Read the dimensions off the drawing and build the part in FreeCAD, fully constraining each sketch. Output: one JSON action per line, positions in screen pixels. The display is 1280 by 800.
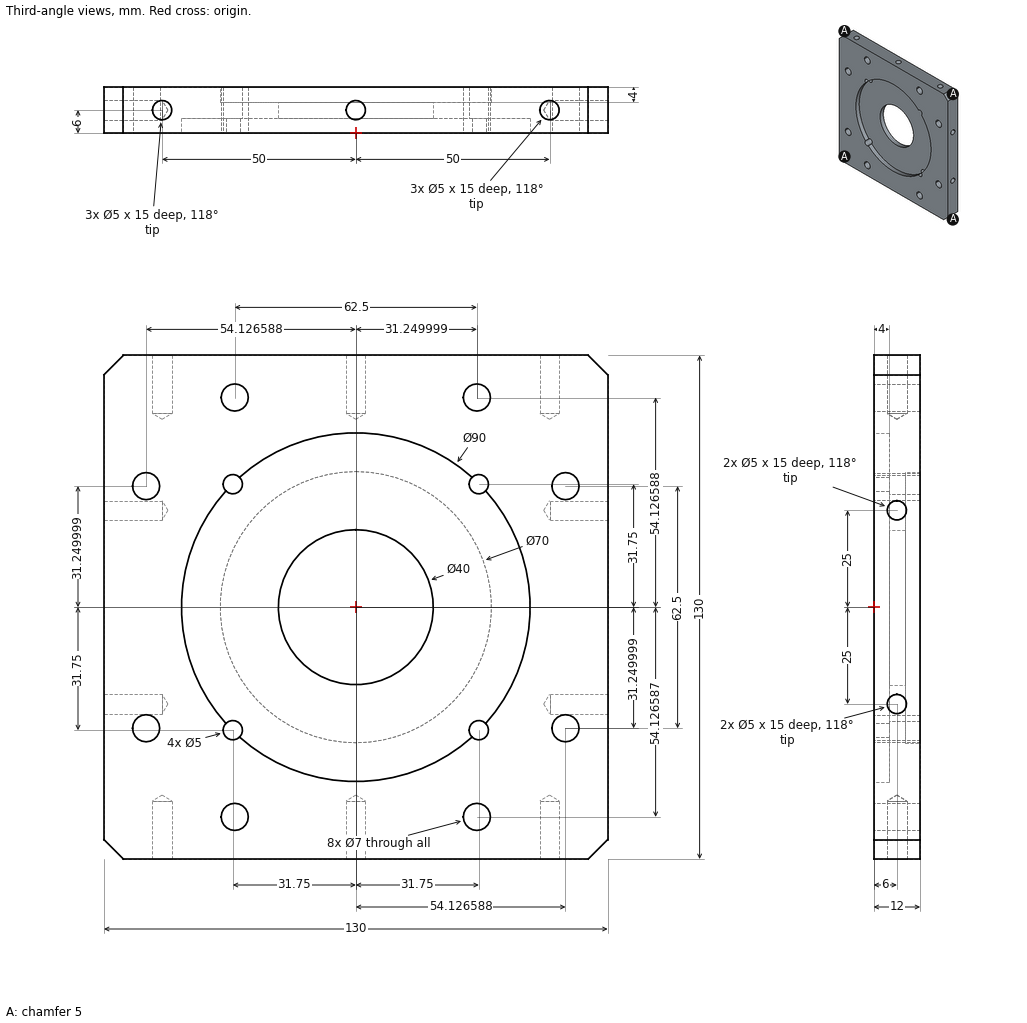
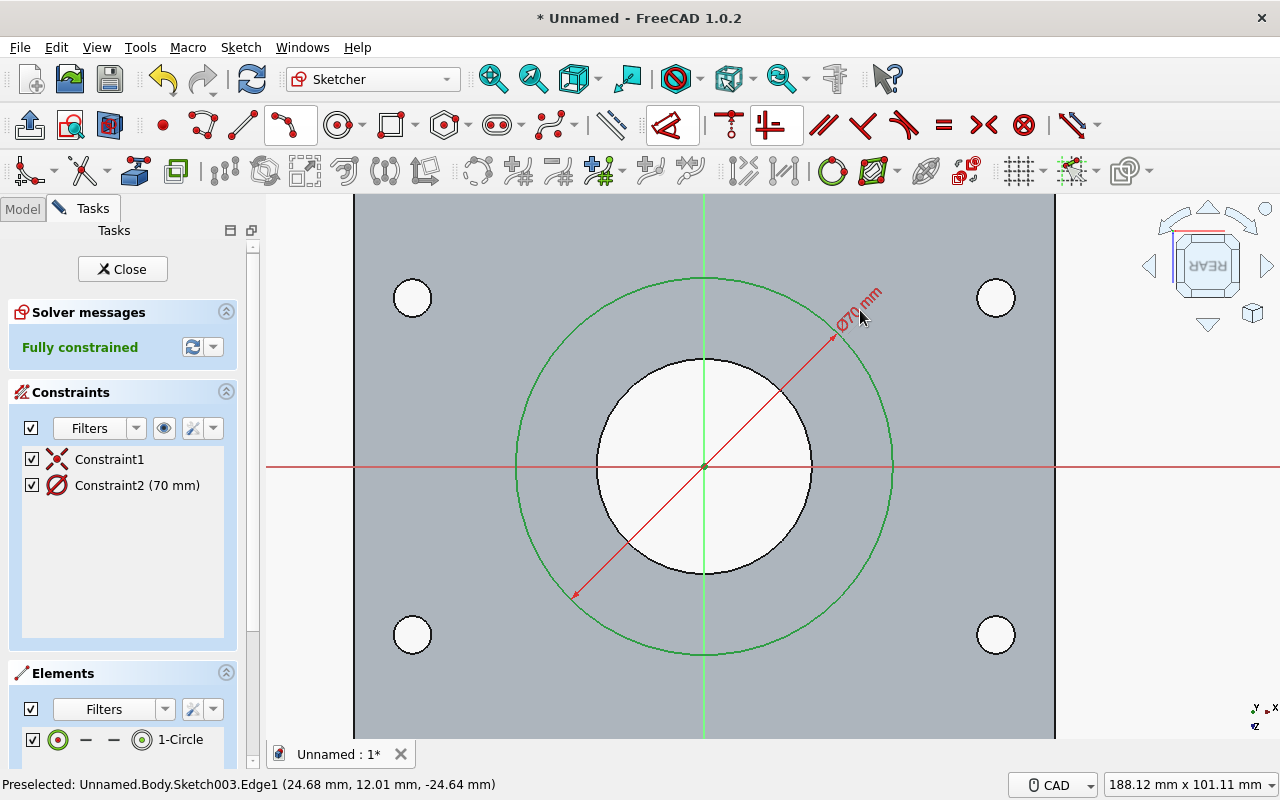
{"action": "left_click", "coordinate": [123, 269]}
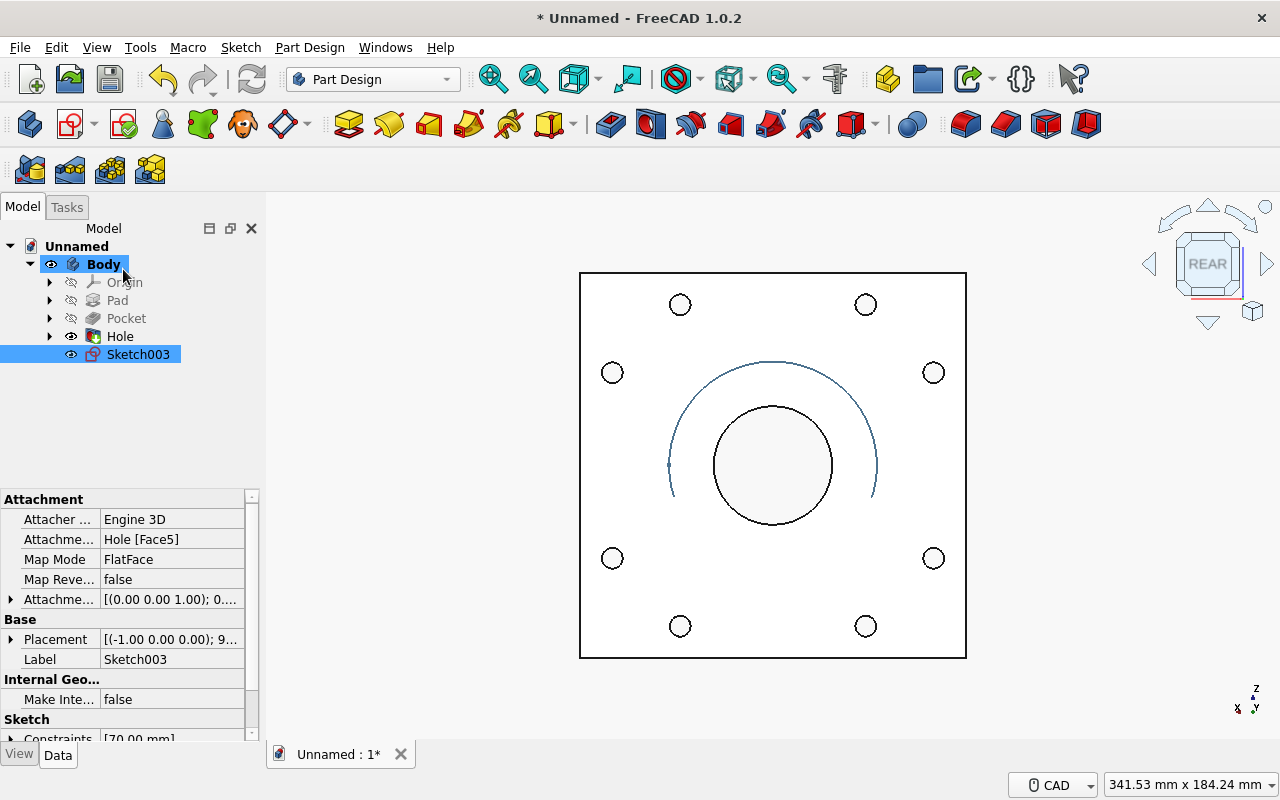
{"action": "left_click", "coordinate": [612, 124]}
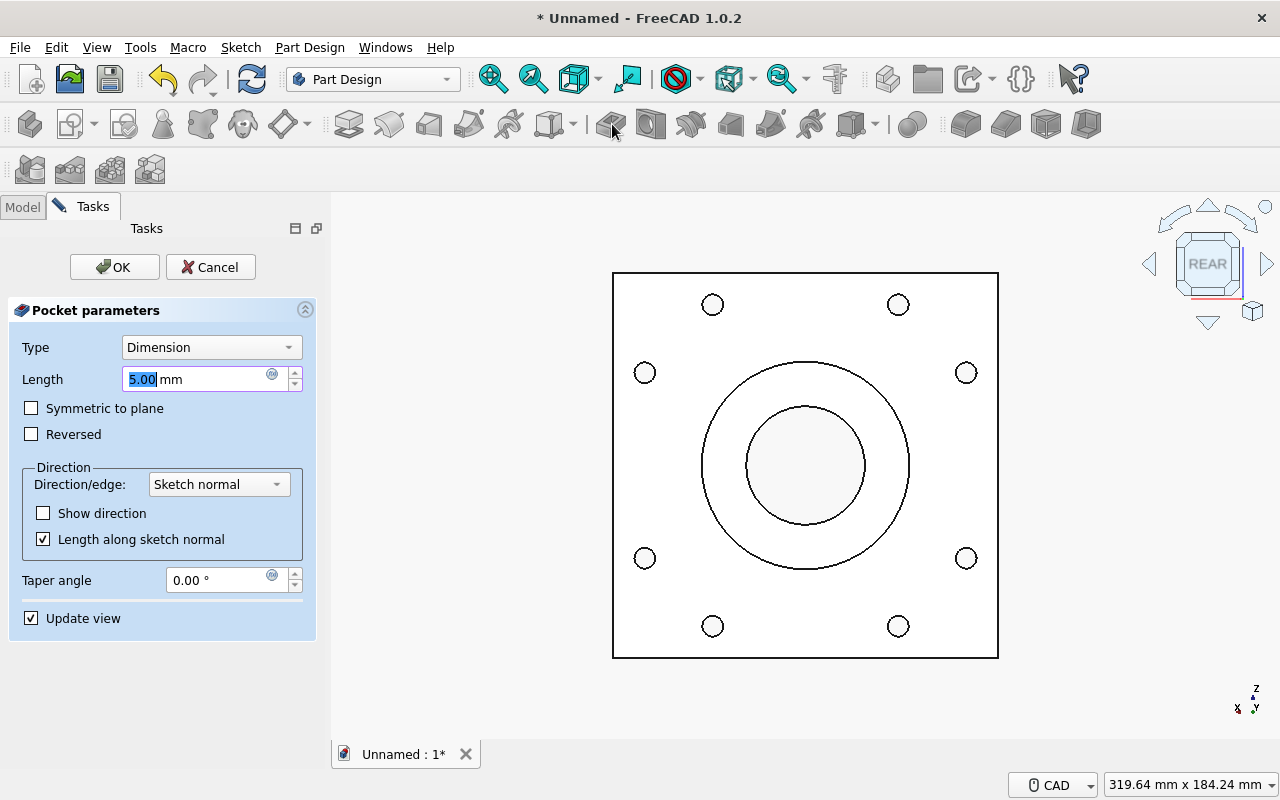
{"action": "type", "text": "4"}
{"action": "key", "text": "Tab"}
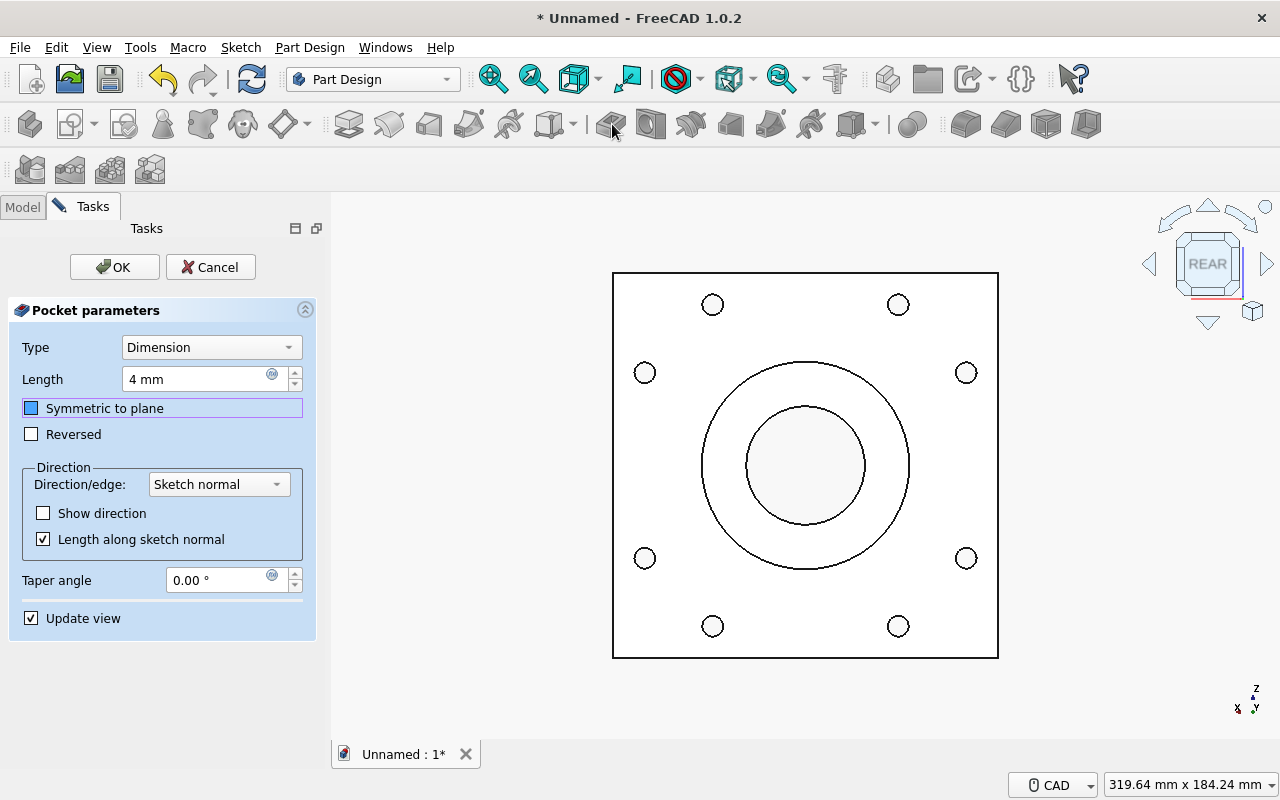
{"action": "left_click", "coordinate": [115, 267]}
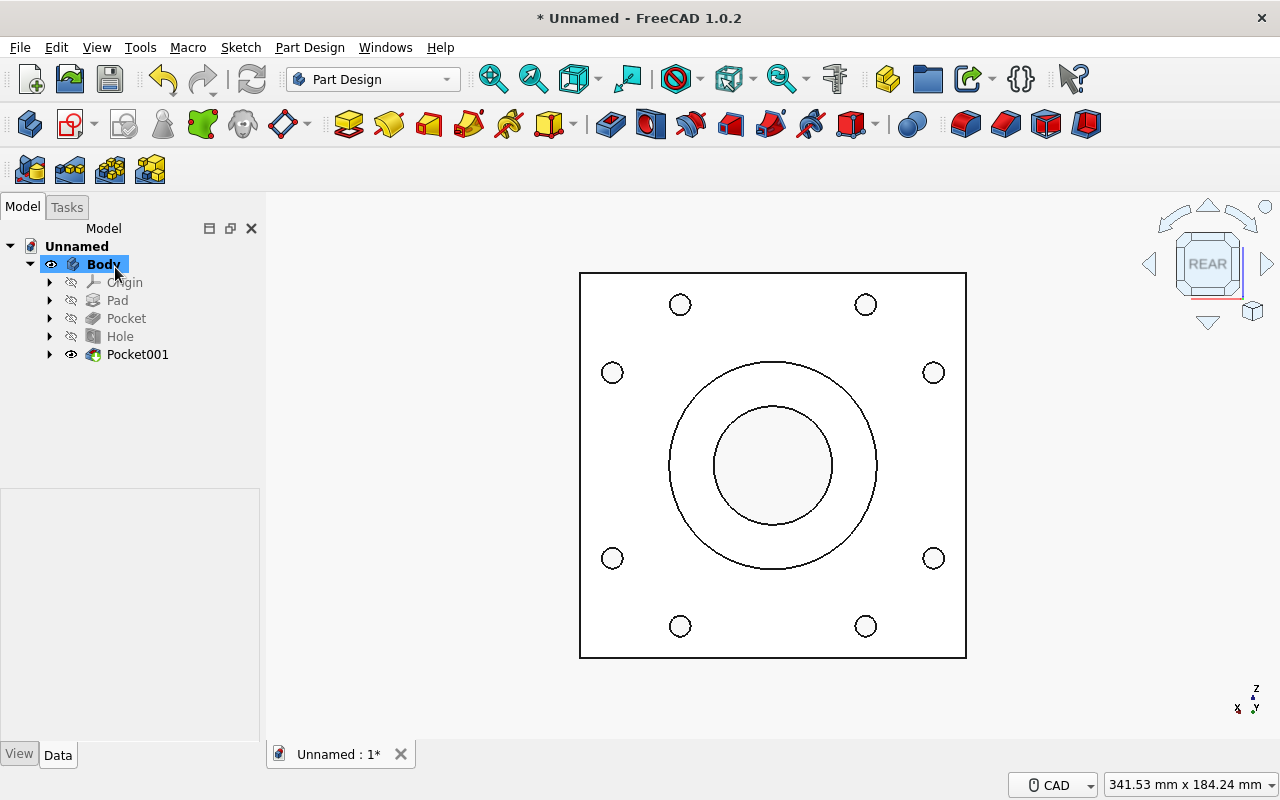
{"action": "key", "text": "0"}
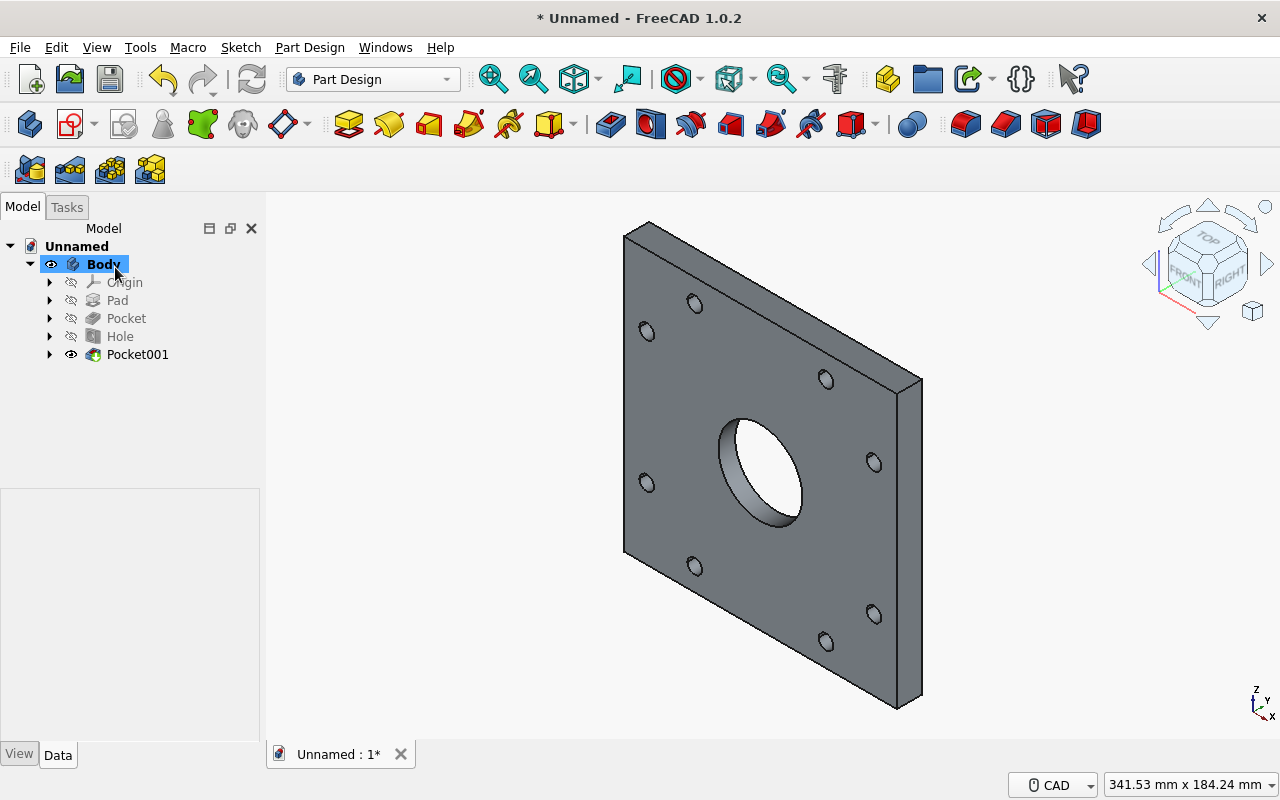
{"action": "left_click", "coordinate": [721, 359]}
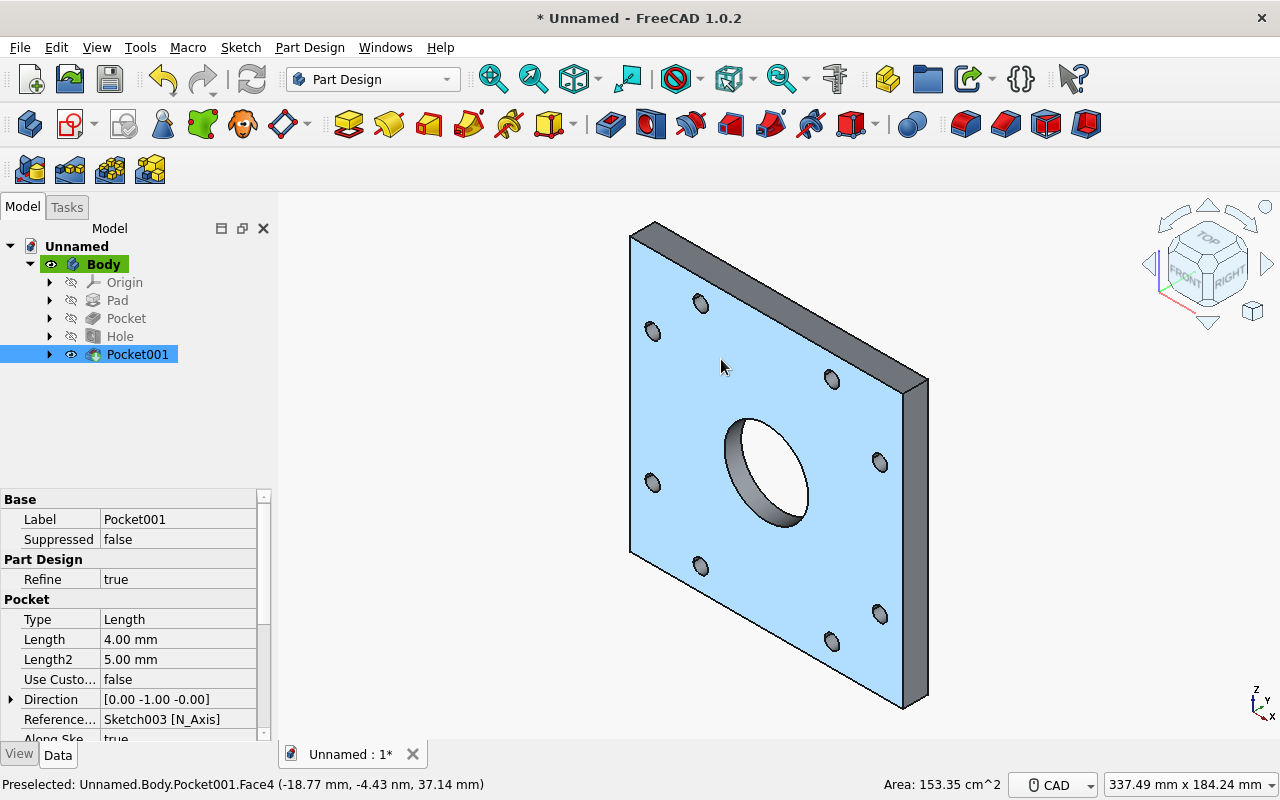
{"action": "left_click", "coordinate": [70, 124]}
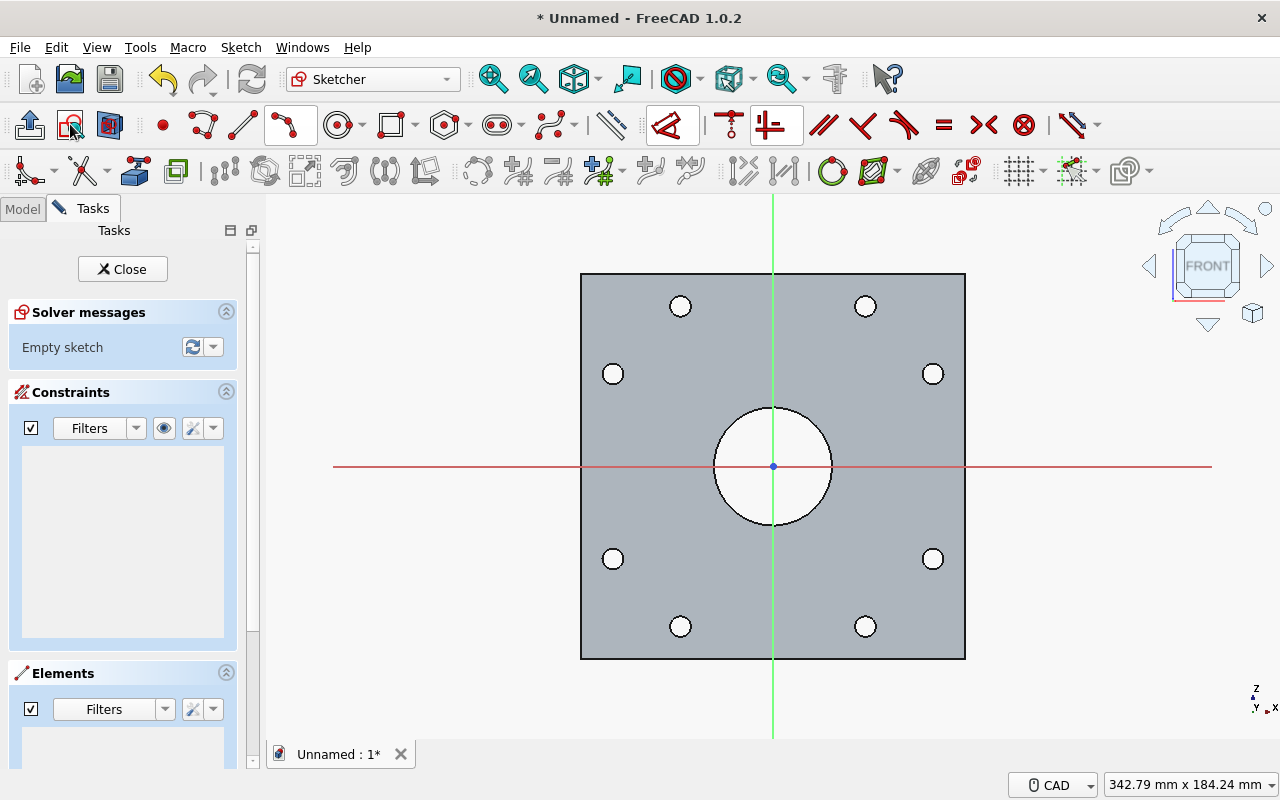
{"action": "key", "text": "g c"}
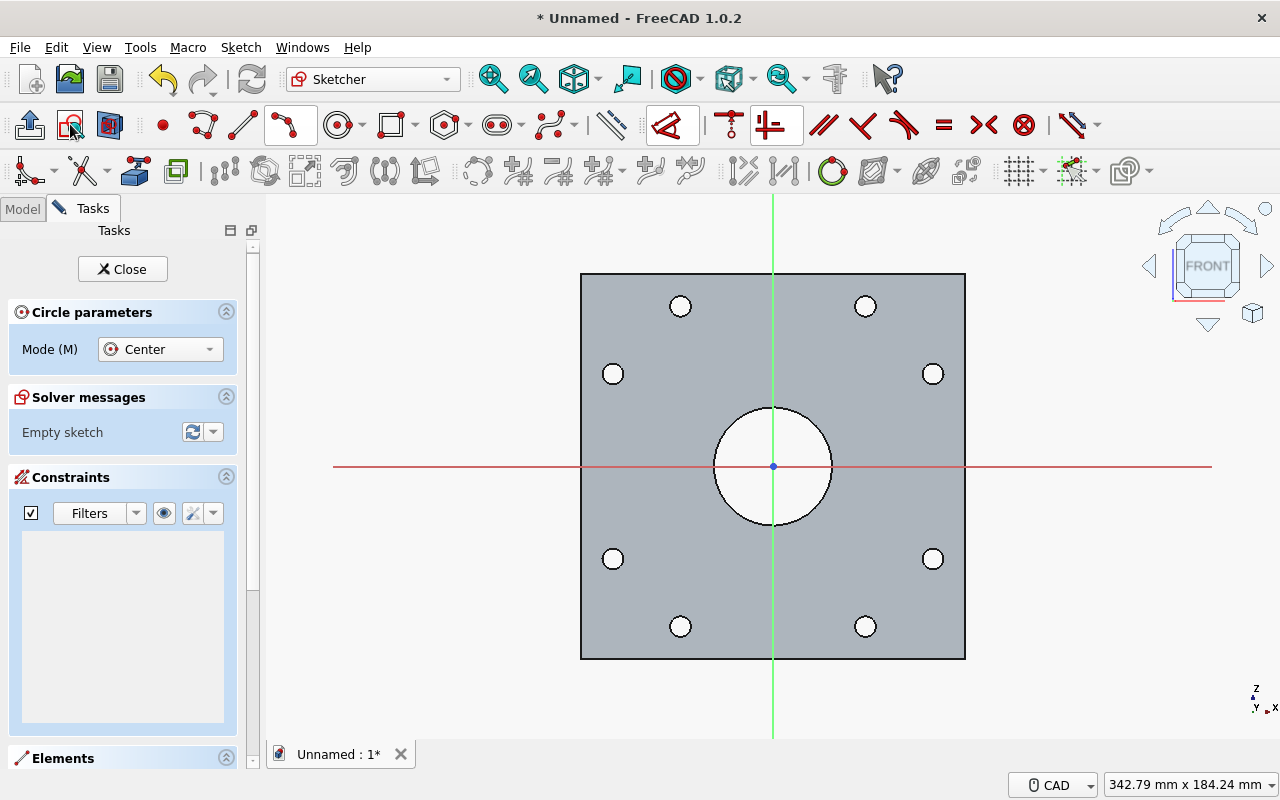
{"action": "left_click", "coordinate": [773, 467]}
{"action": "left_click", "coordinate": [867, 372]}
{"action": "key", "text": "Escape"}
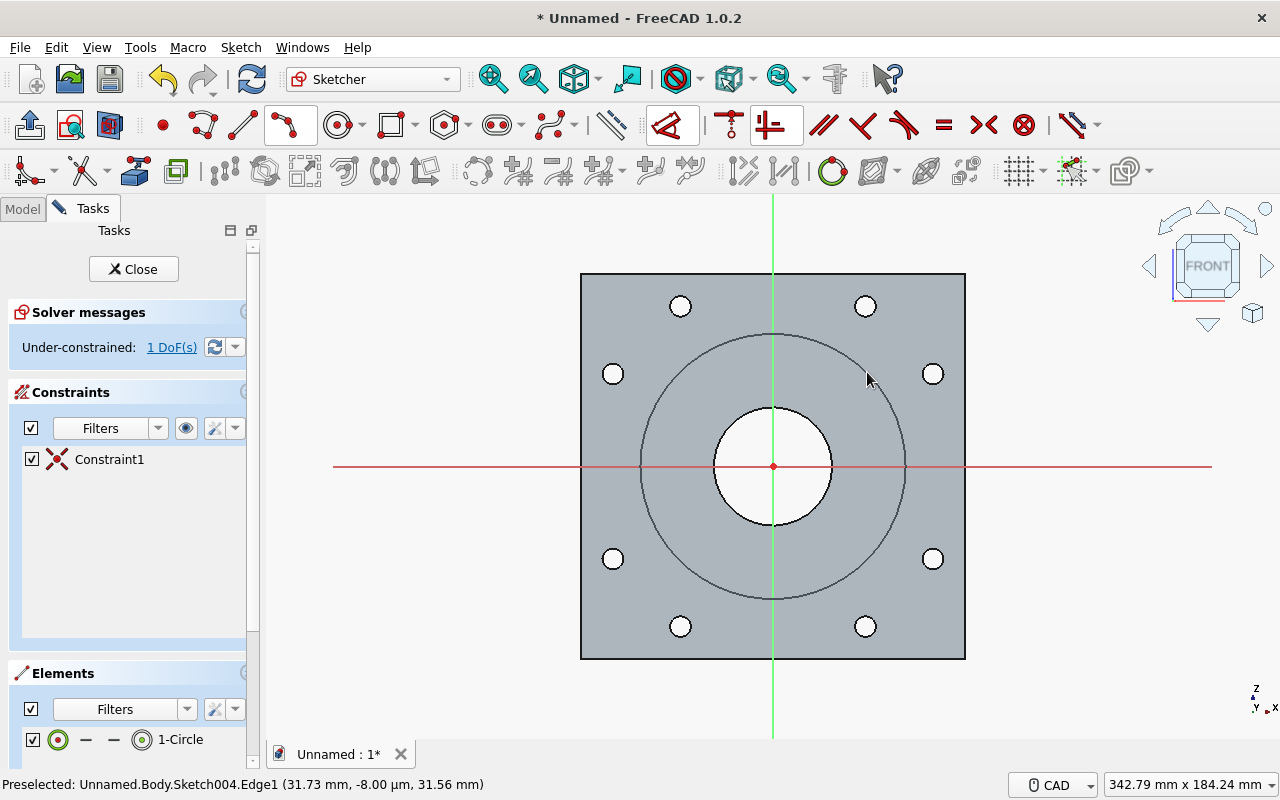
{"action": "key", "text": "d"}